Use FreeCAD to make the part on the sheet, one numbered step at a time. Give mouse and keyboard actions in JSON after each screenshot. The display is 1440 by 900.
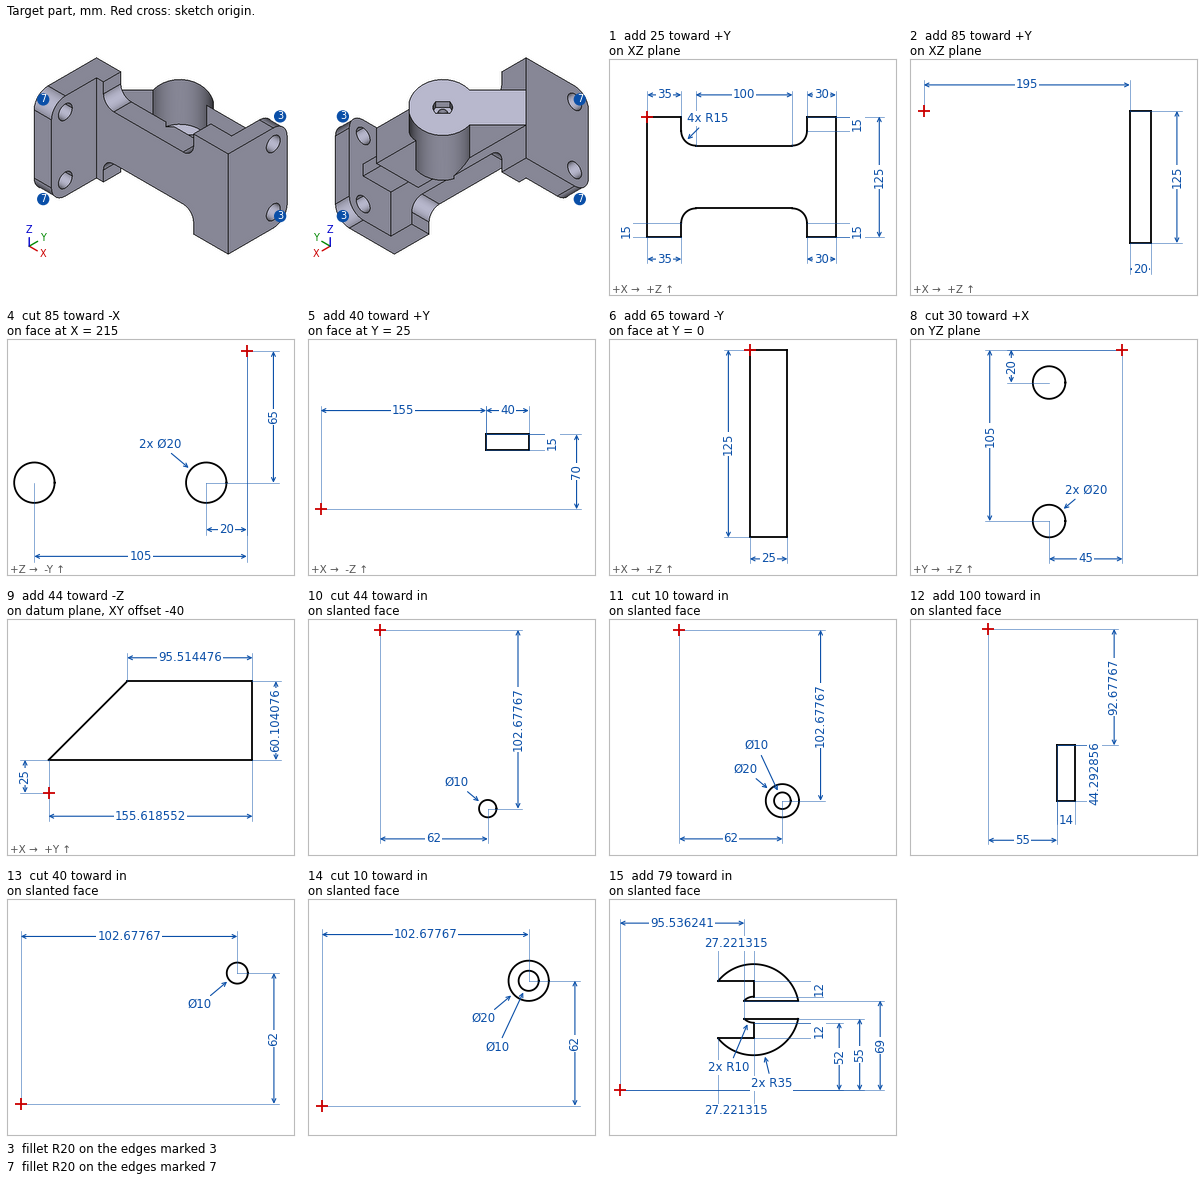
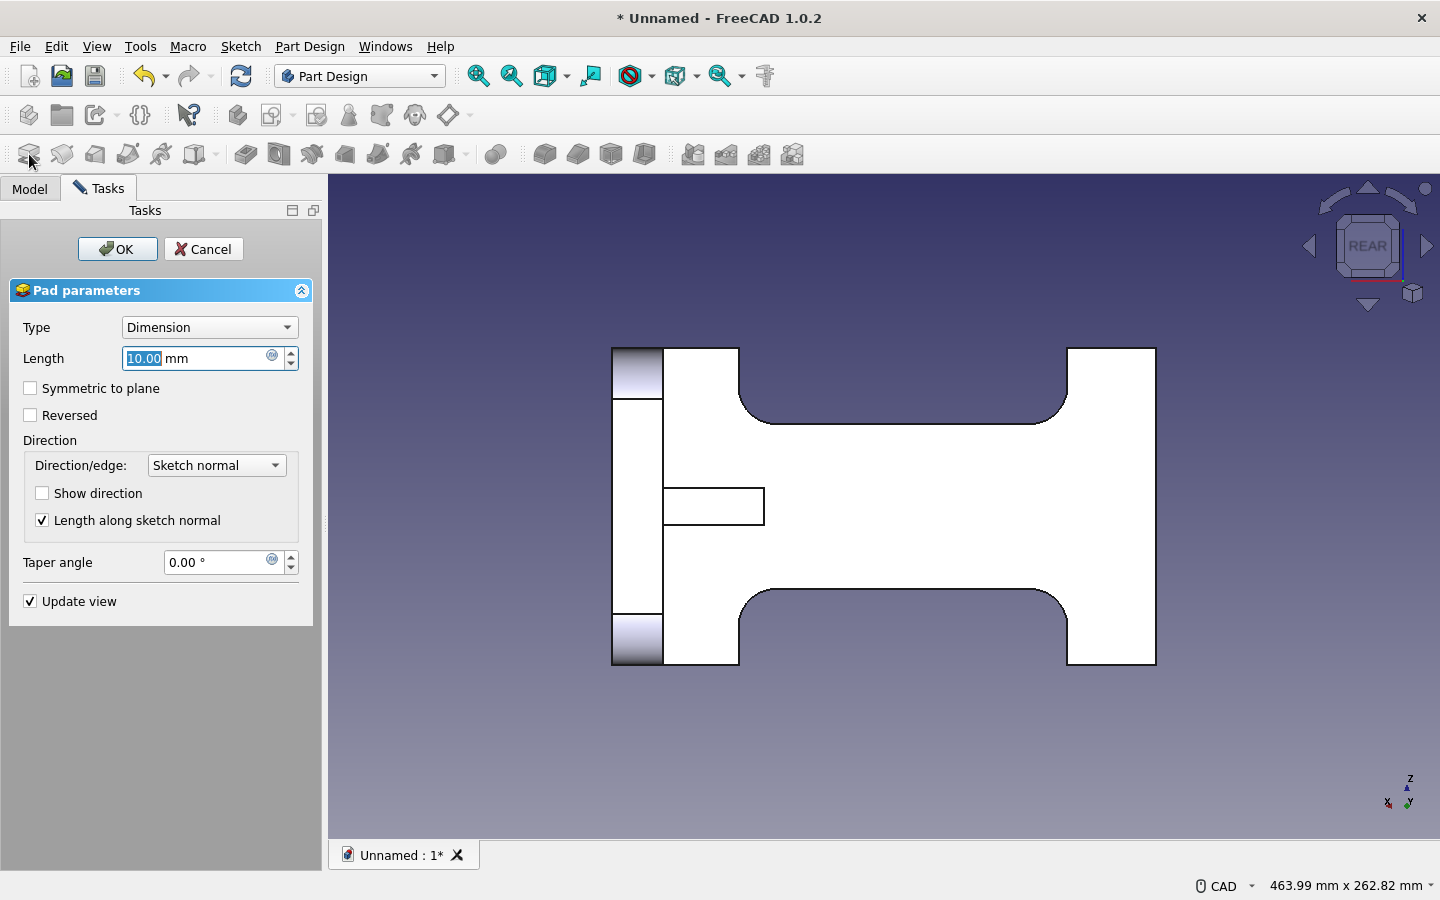
{"action": "type", "text": "40"}
{"action": "key", "text": "Tab"}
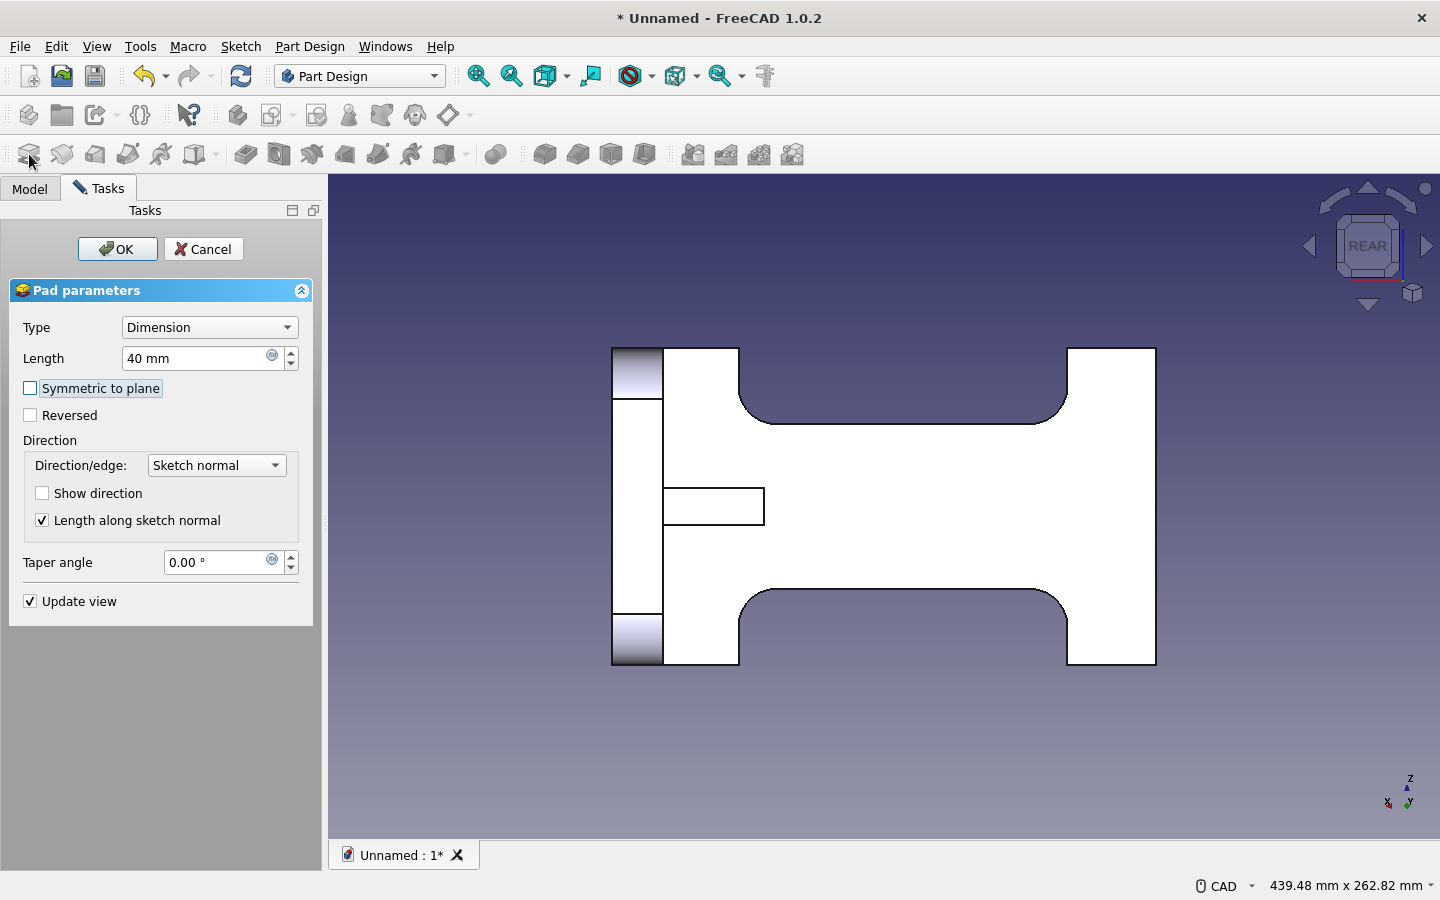
{"action": "left_click", "coordinate": [118, 249]}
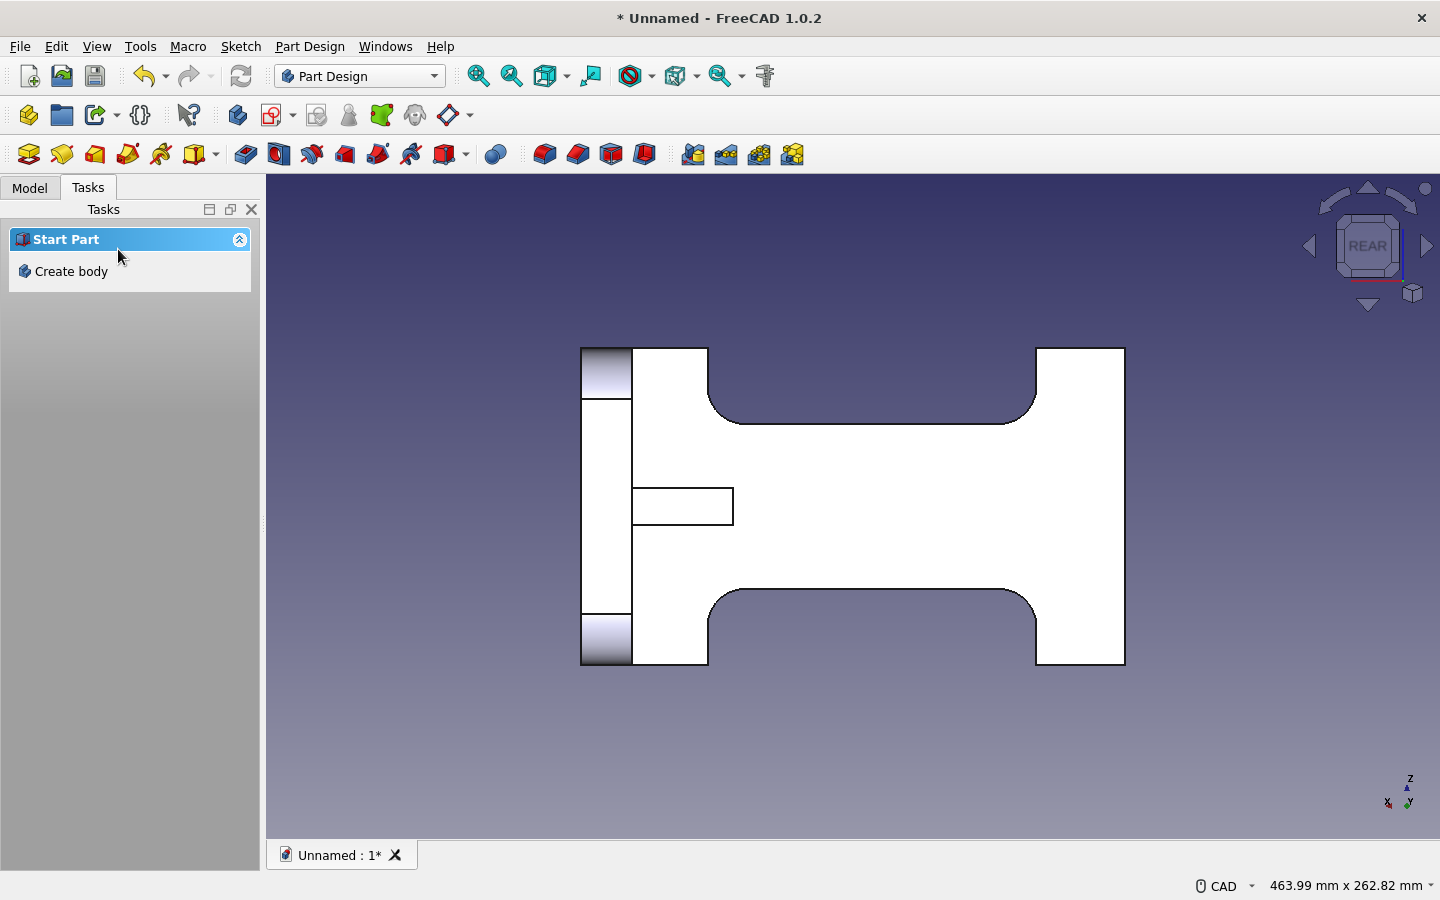
{"action": "key", "text": "0"}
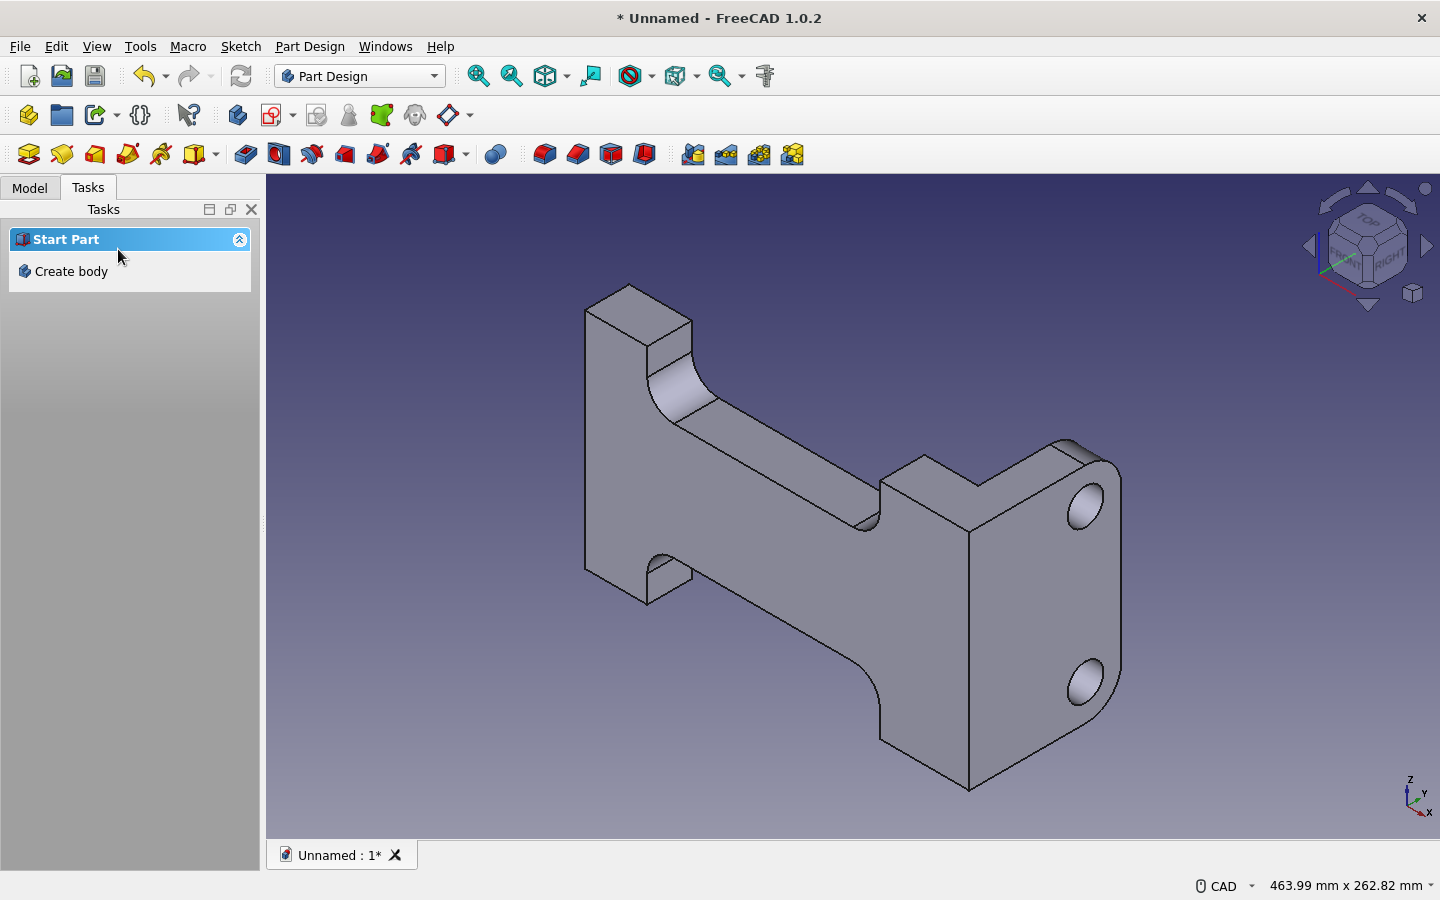
{"action": "left_click", "coordinate": [887, 613]}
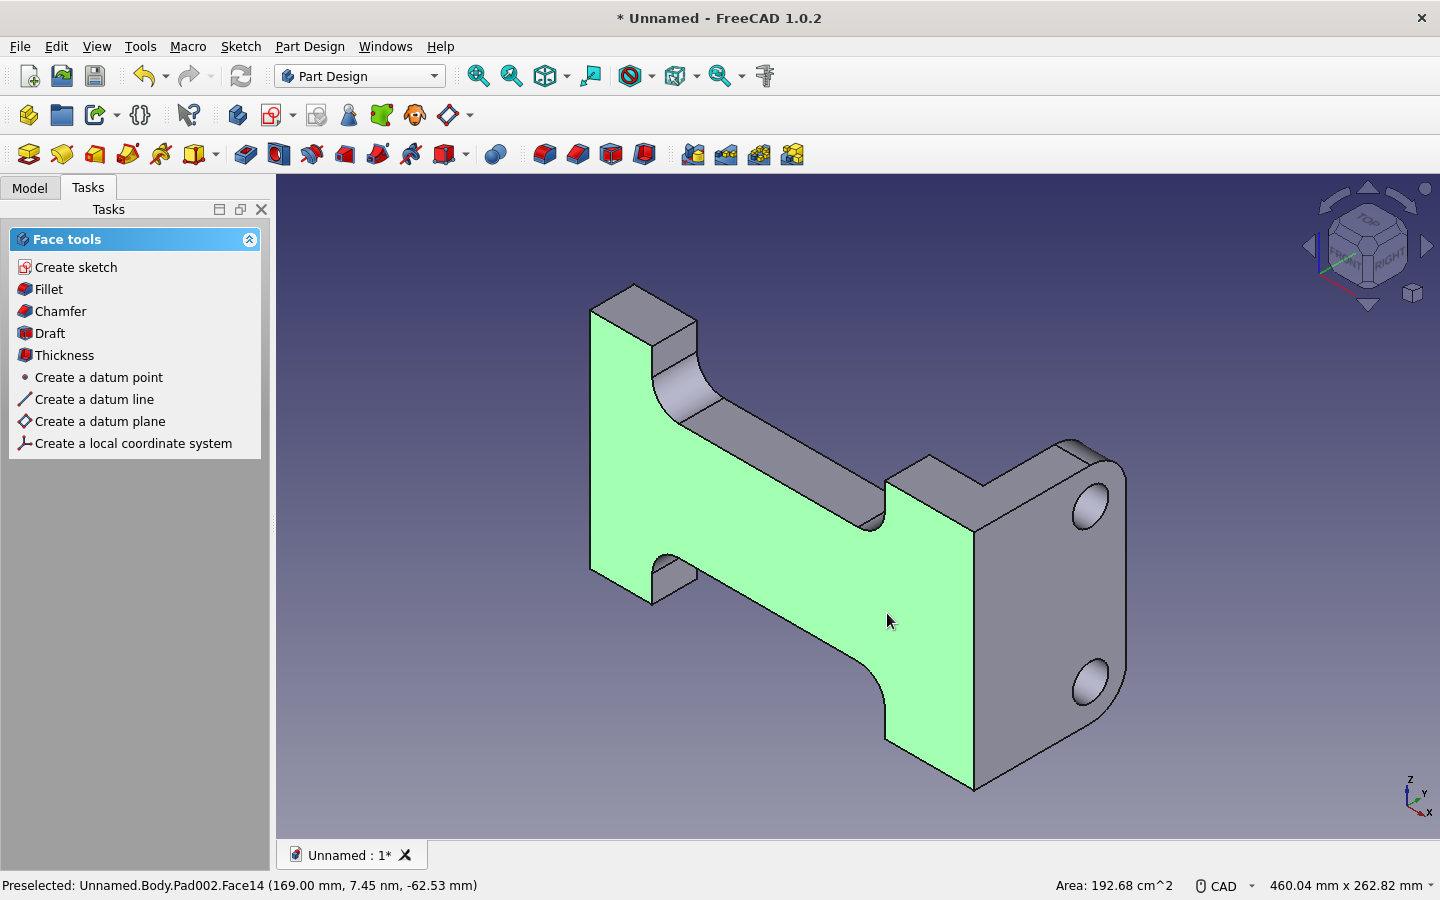
{"action": "left_click", "coordinate": [270, 116]}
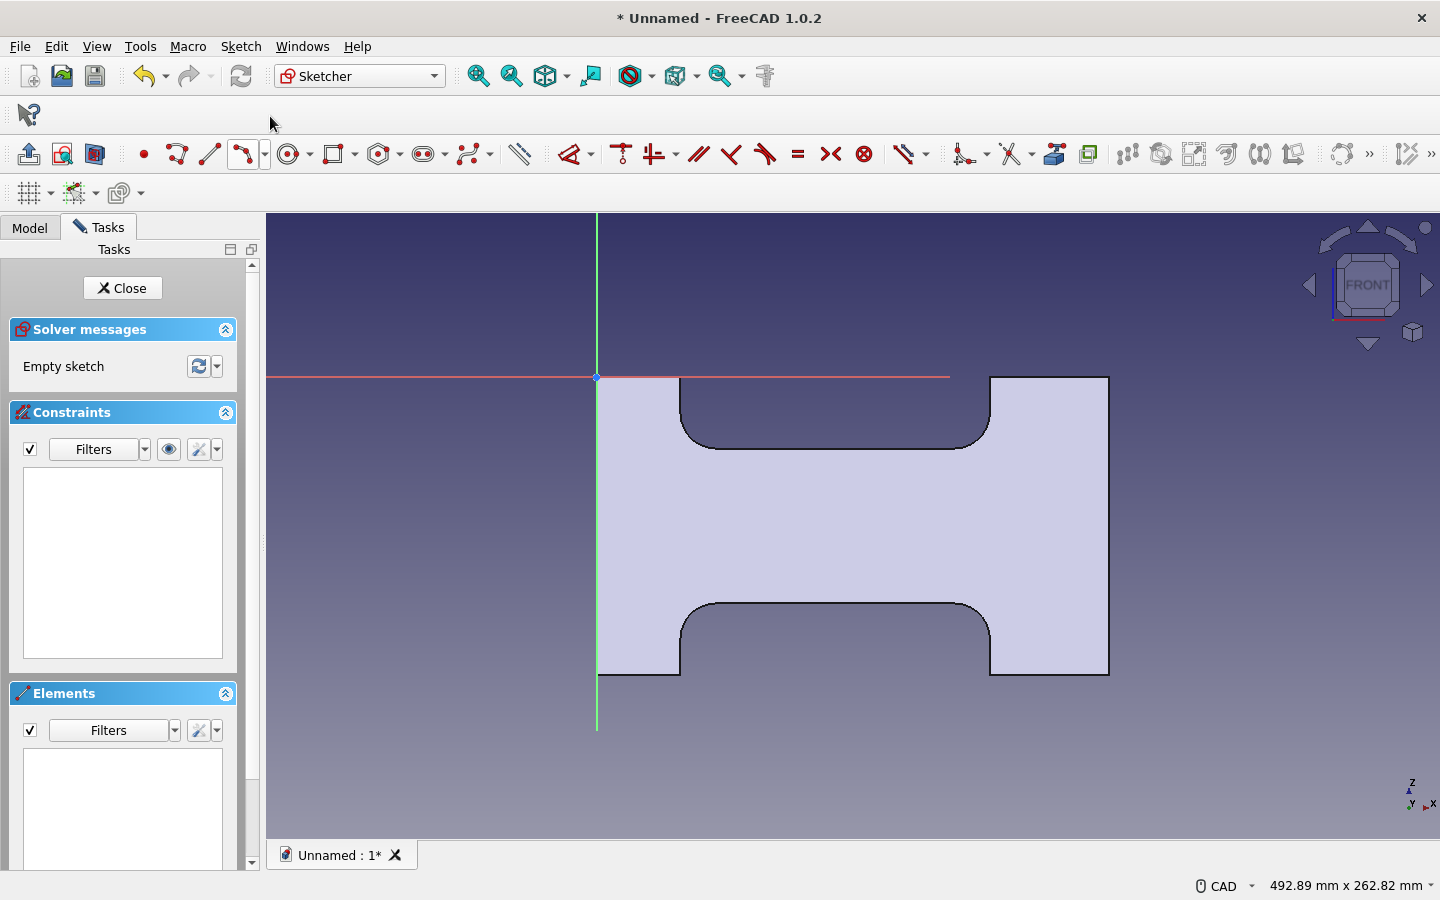
{"action": "scroll", "coordinate": [306, 526], "scroll_direction": "up", "scroll_amount": 2}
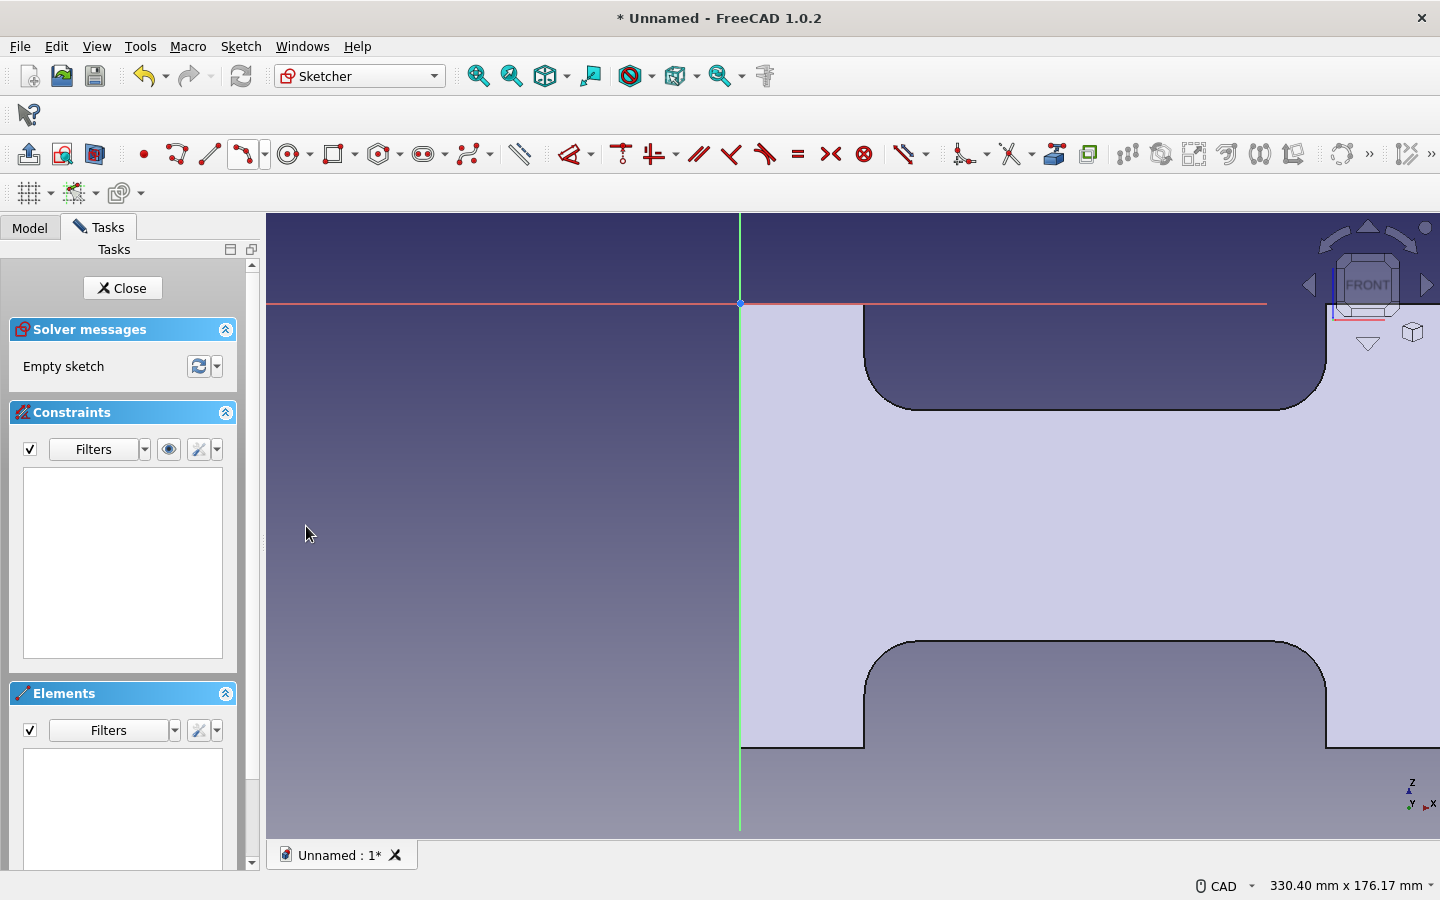
{"action": "key", "text": "g r"}